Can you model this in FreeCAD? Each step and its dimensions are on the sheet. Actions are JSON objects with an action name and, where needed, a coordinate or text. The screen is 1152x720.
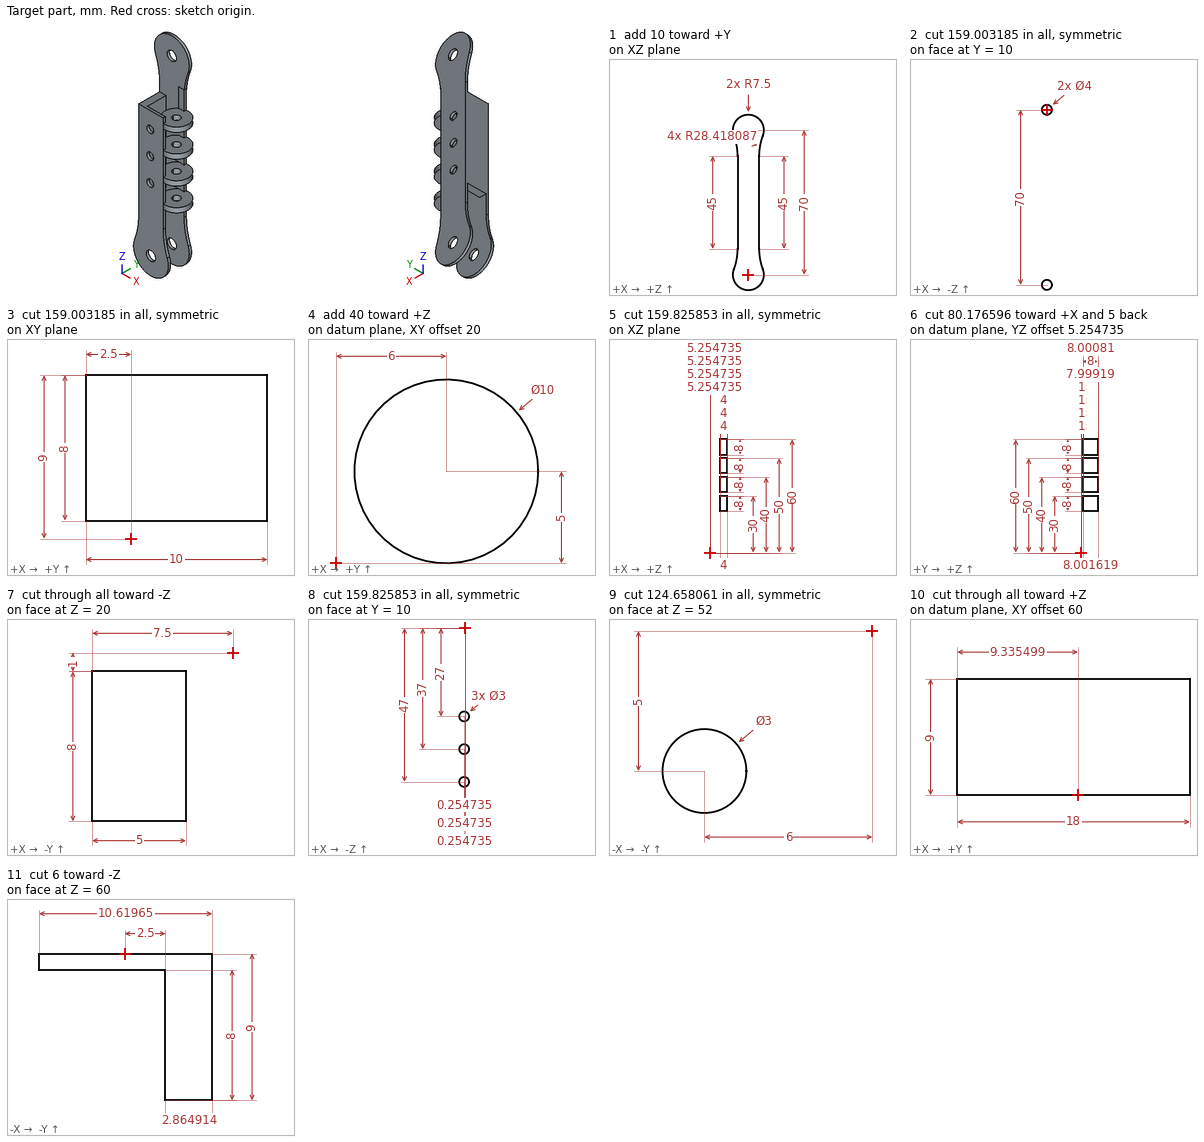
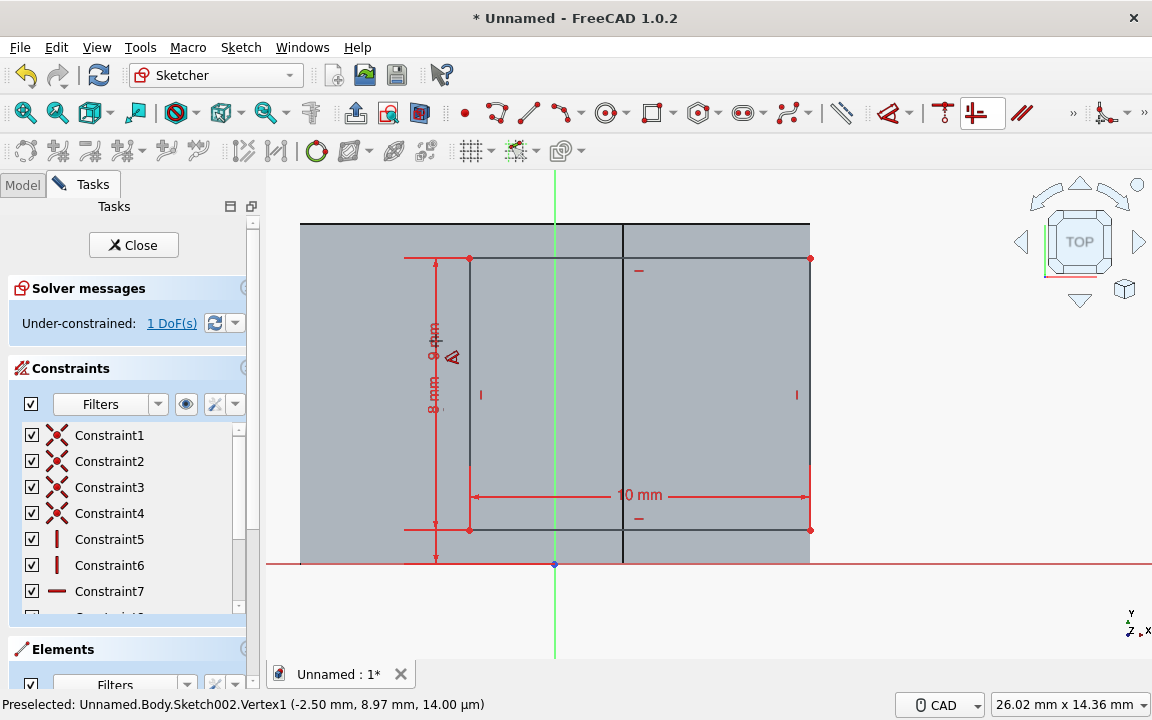
{"action": "left_click", "coordinate": [470, 258]}
{"action": "left_click", "coordinate": [512, 598]}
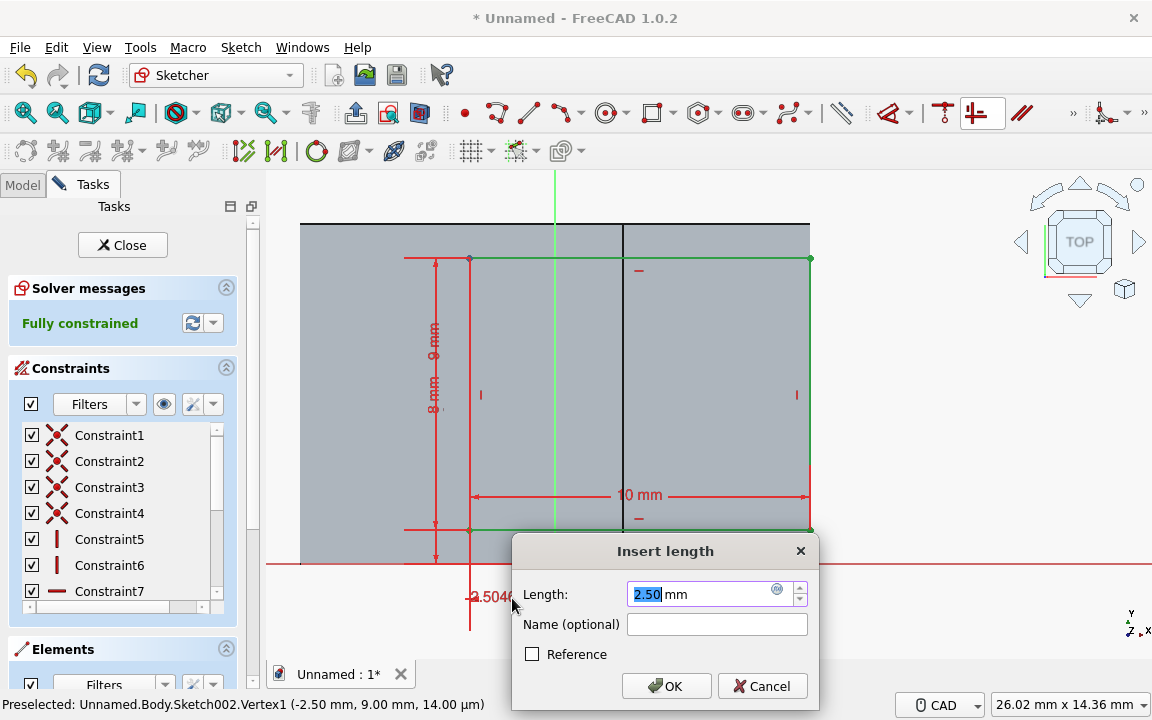
{"action": "type", "text": "2.5"}
{"action": "key", "text": "Return"}
{"action": "key", "text": "Escape"}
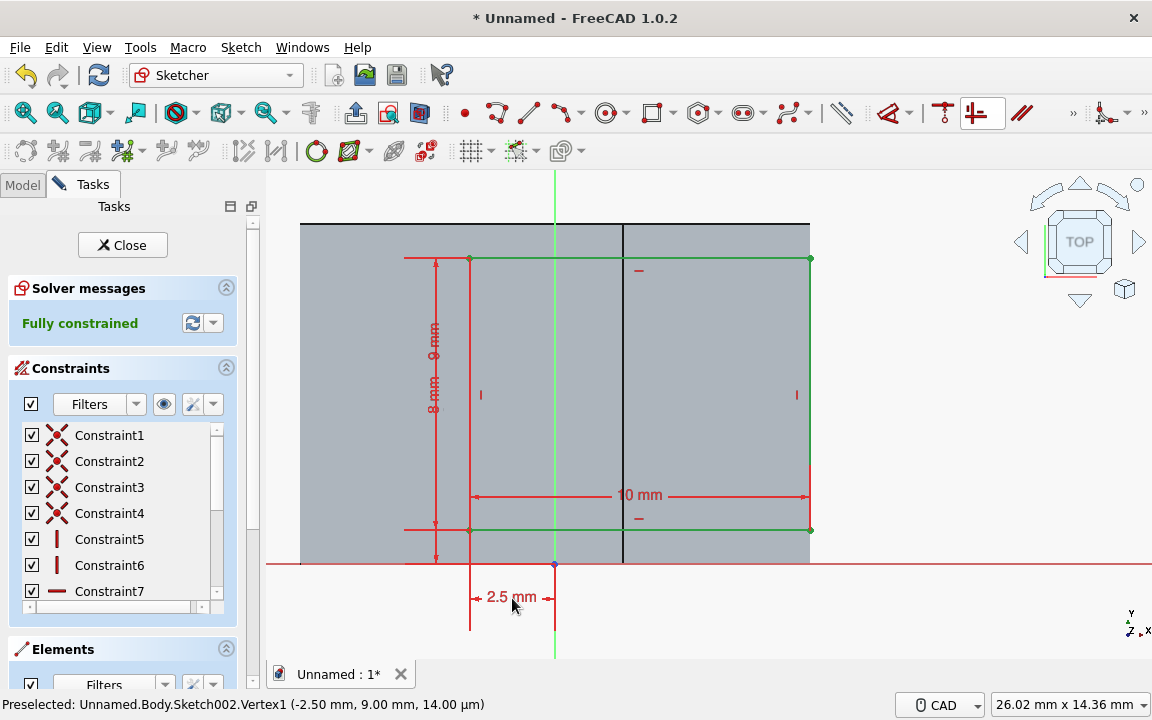
{"action": "left_click", "coordinate": [123, 245]}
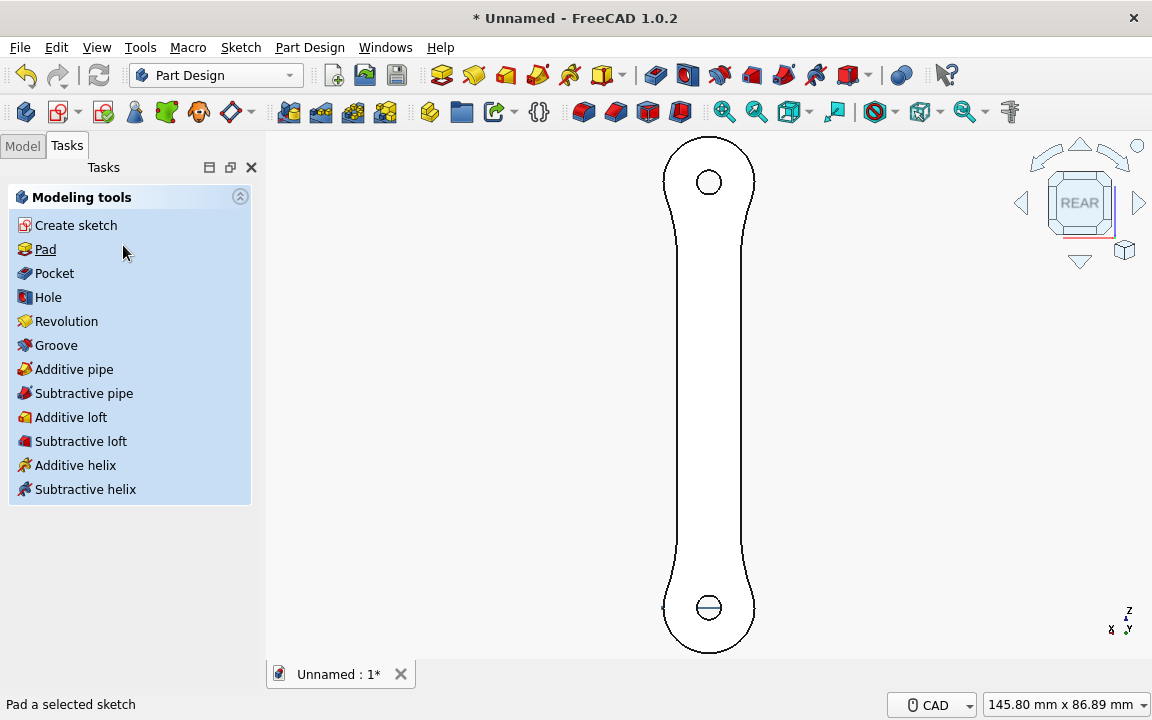
{"action": "left_click", "coordinate": [656, 76]}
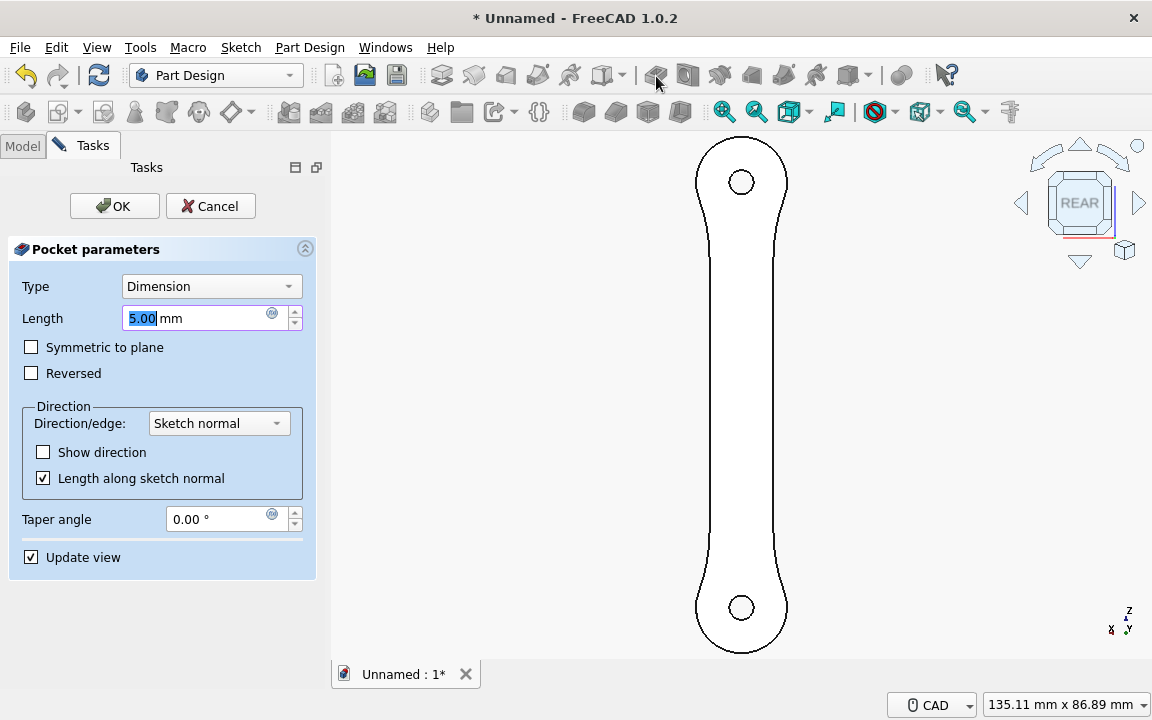
{"action": "type", "text": "159.003185"}
{"action": "key", "text": "Tab"}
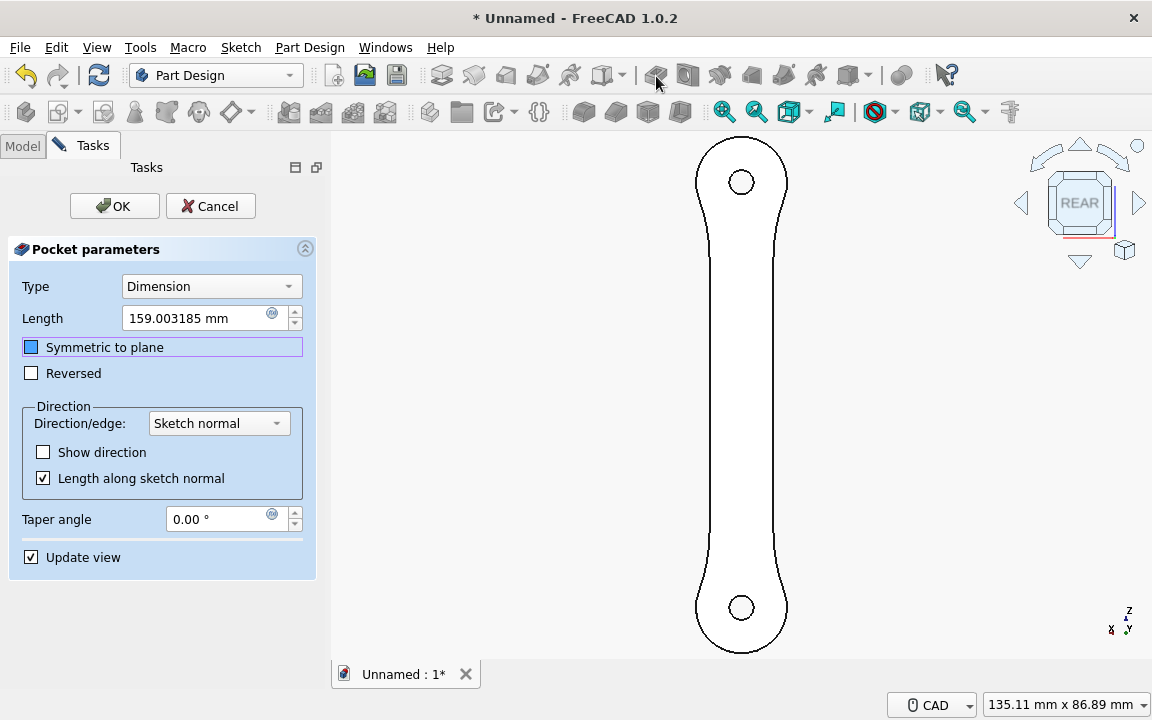
{"action": "left_click", "coordinate": [30, 347]}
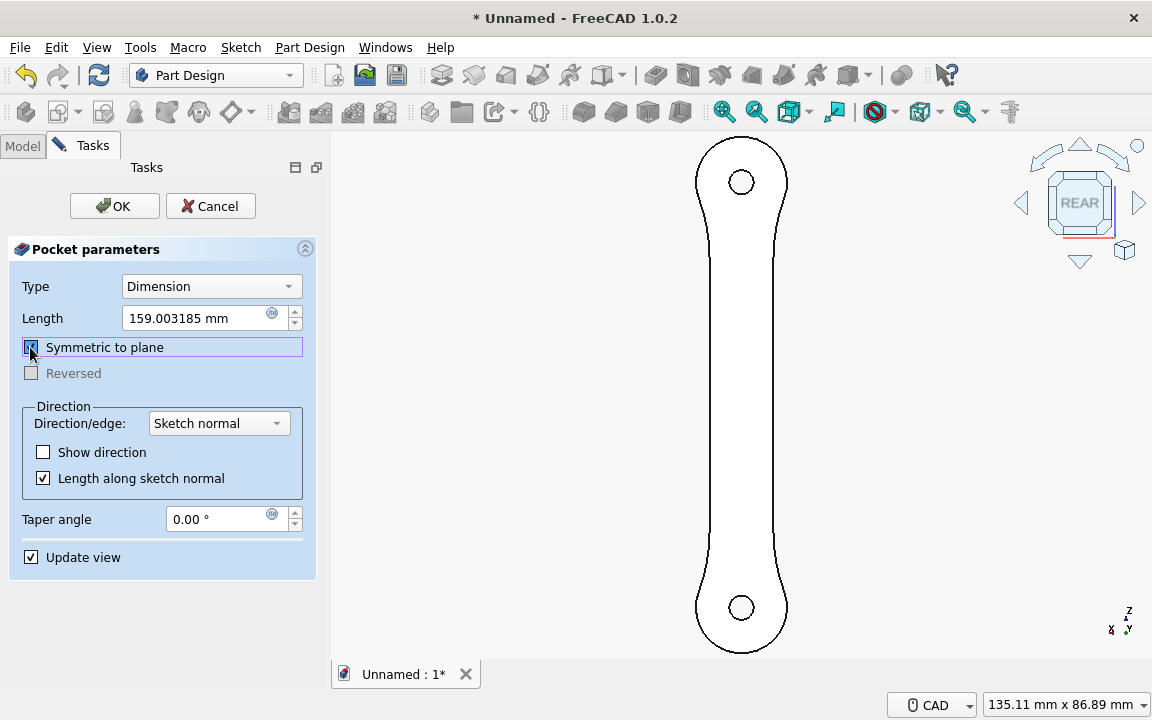
{"action": "left_click", "coordinate": [115, 206]}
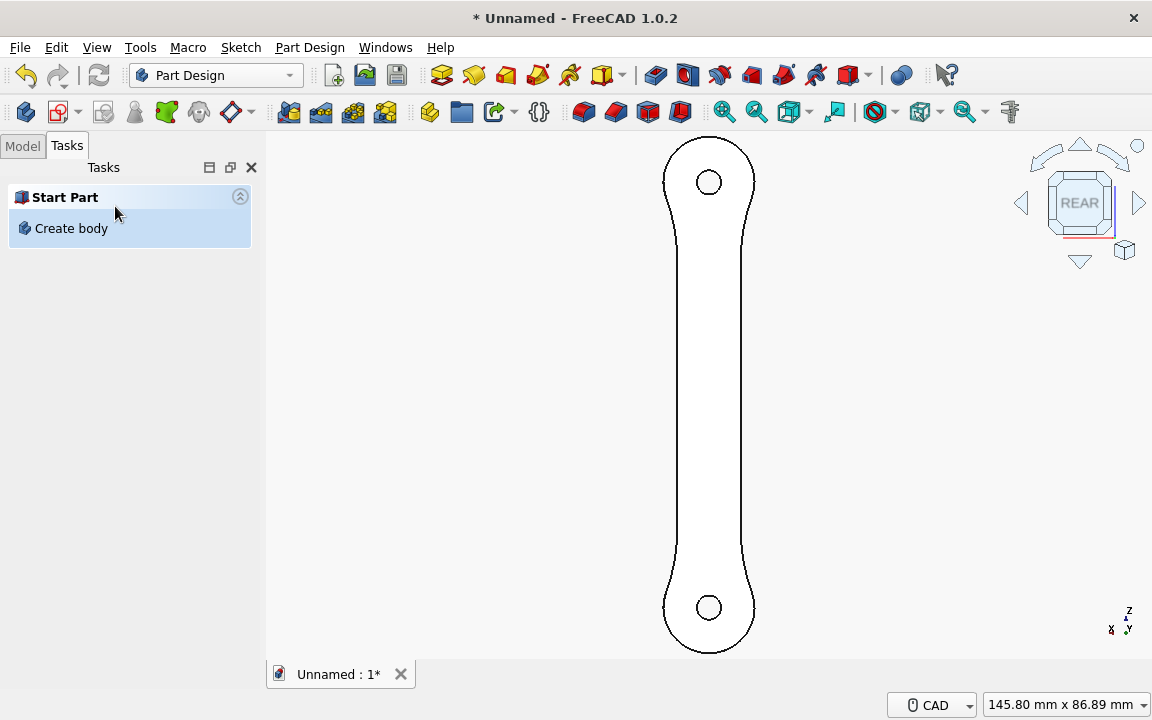
{"action": "left_click", "coordinate": [23, 145]}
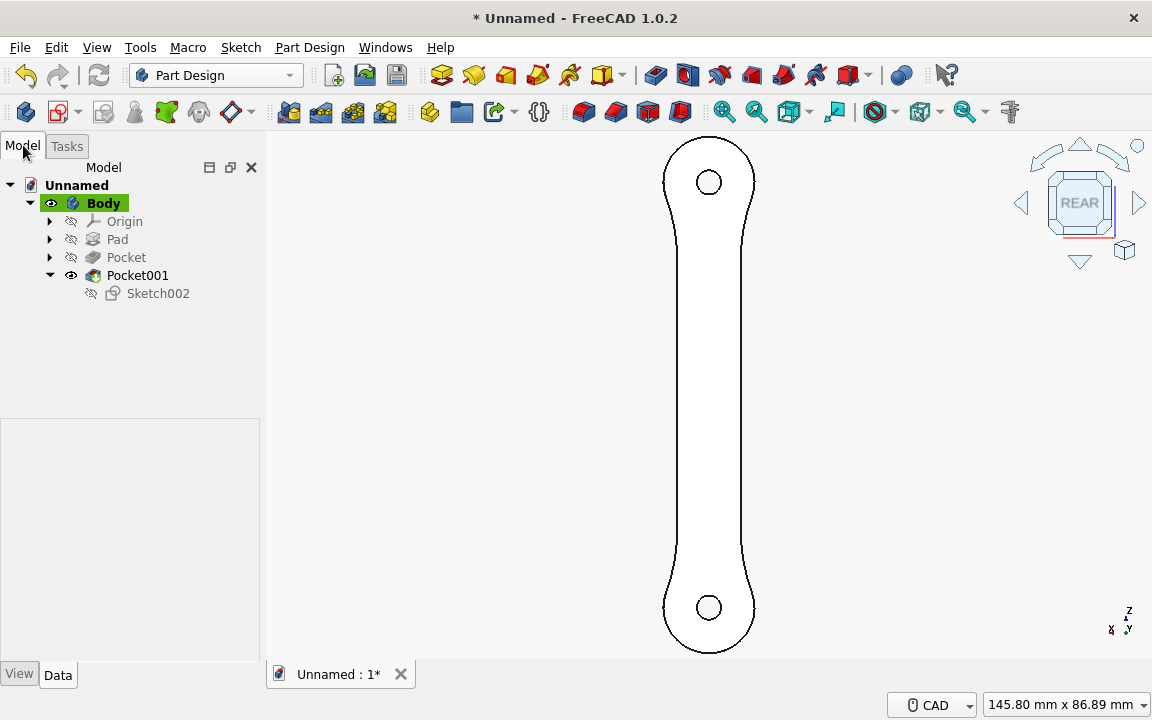
{"action": "left_click", "coordinate": [50, 221]}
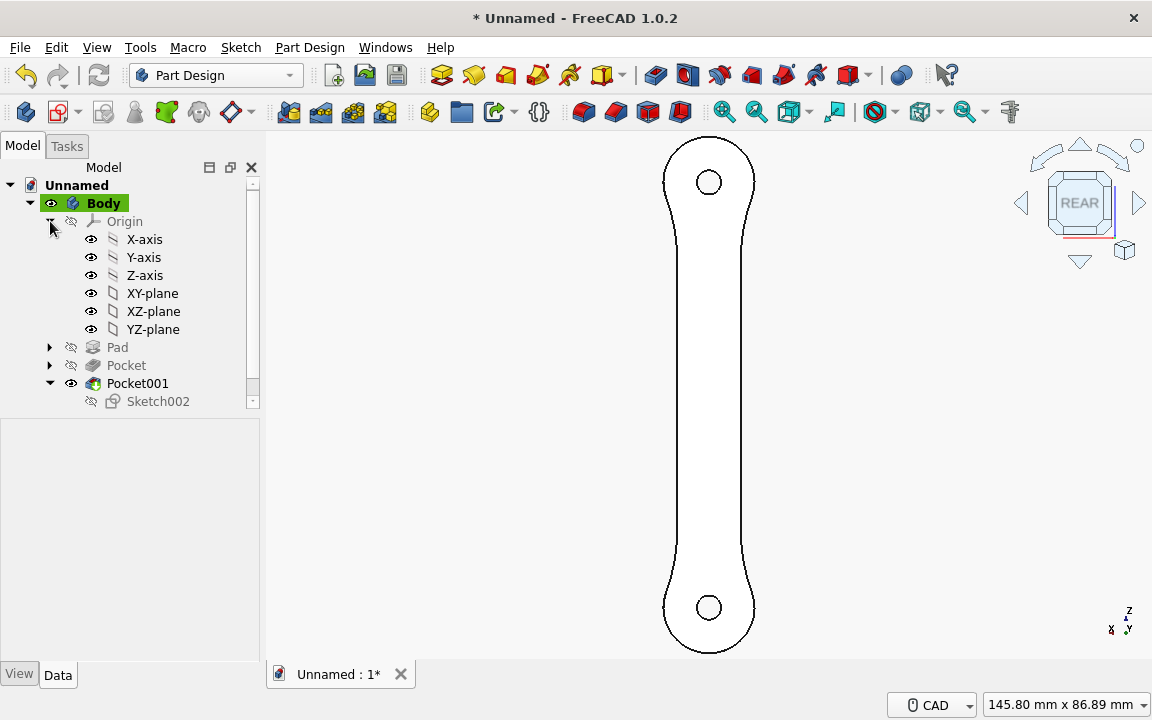
{"action": "left_click", "coordinate": [136, 293]}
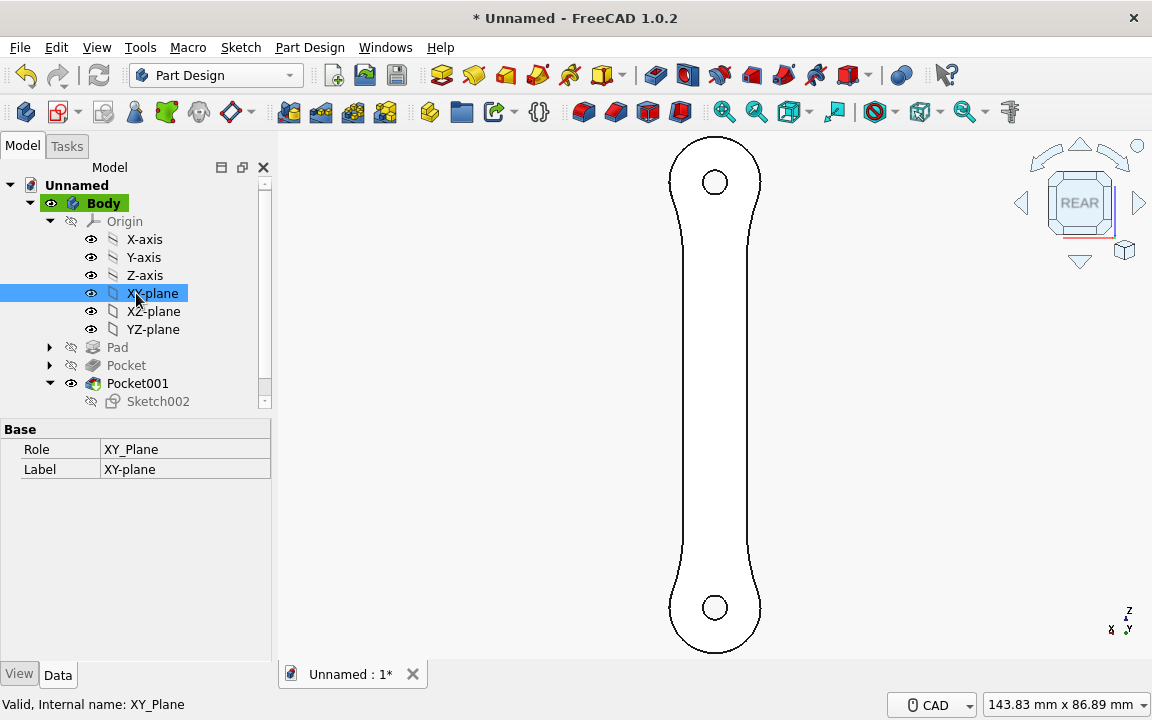
{"action": "left_click", "coordinate": [232, 112]}